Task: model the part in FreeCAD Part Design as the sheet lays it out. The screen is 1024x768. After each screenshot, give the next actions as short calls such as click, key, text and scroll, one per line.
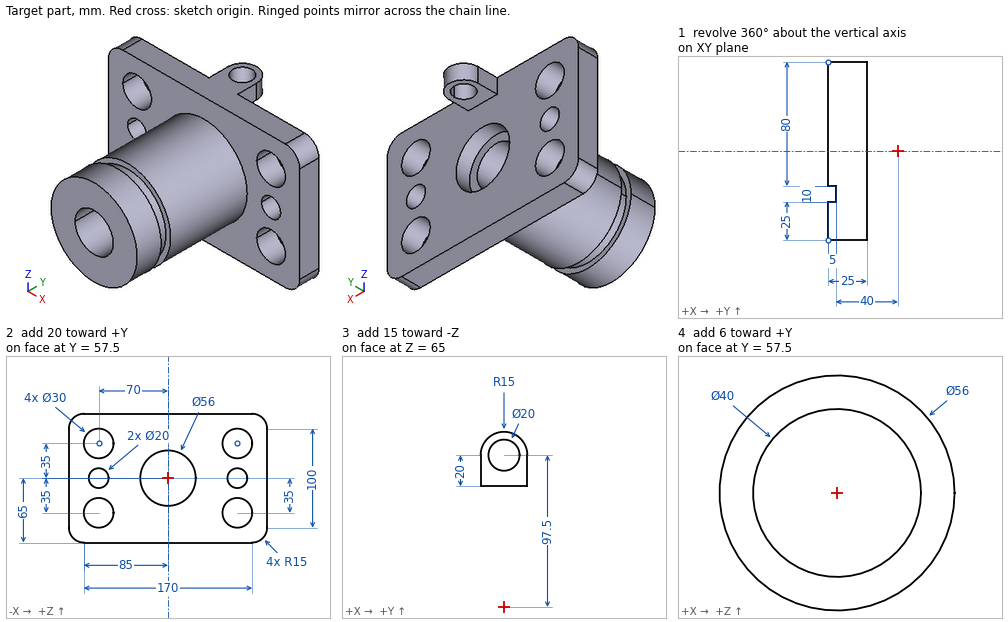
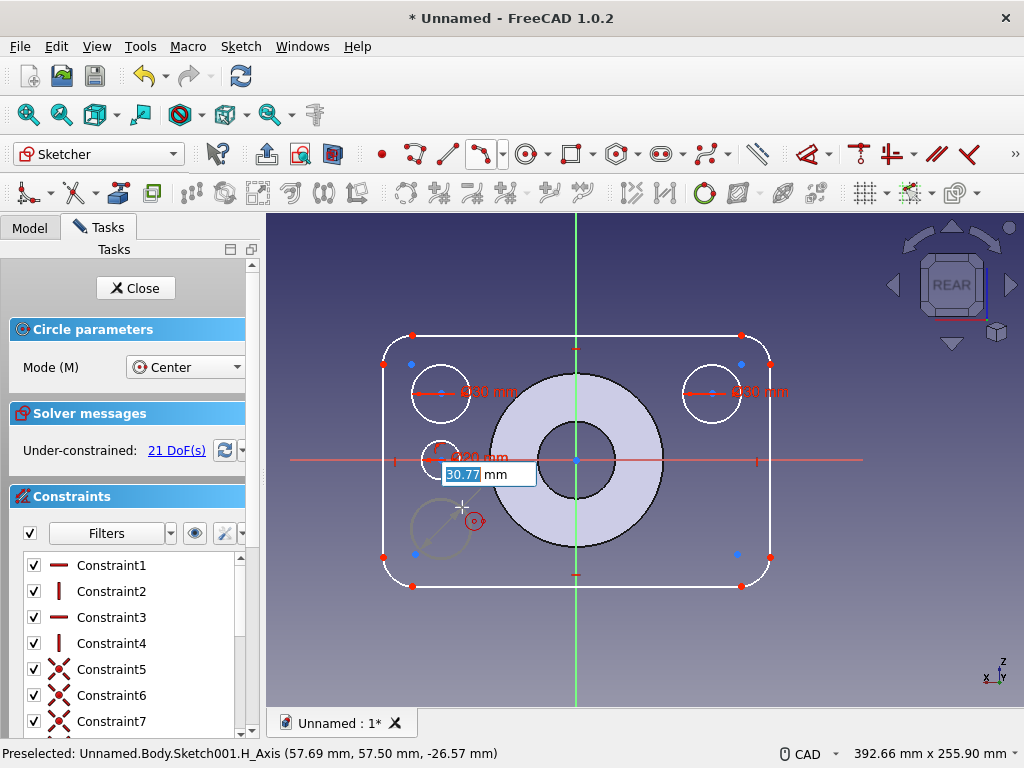
text(30)
key(Return)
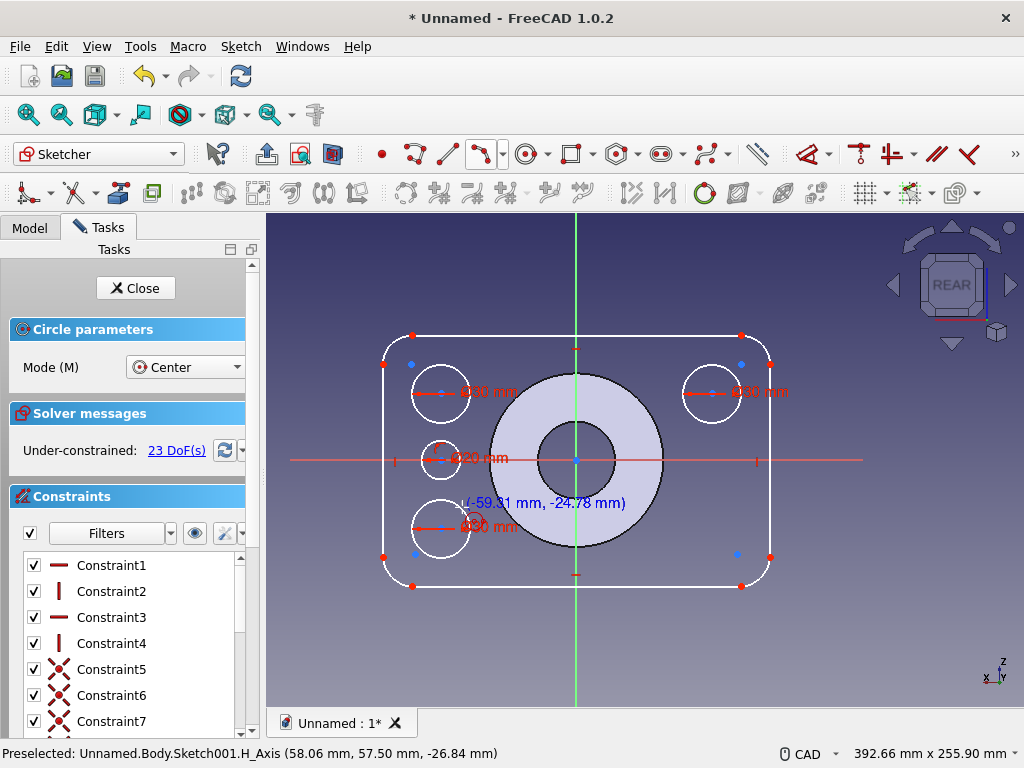
click(712, 460)
move(718, 442)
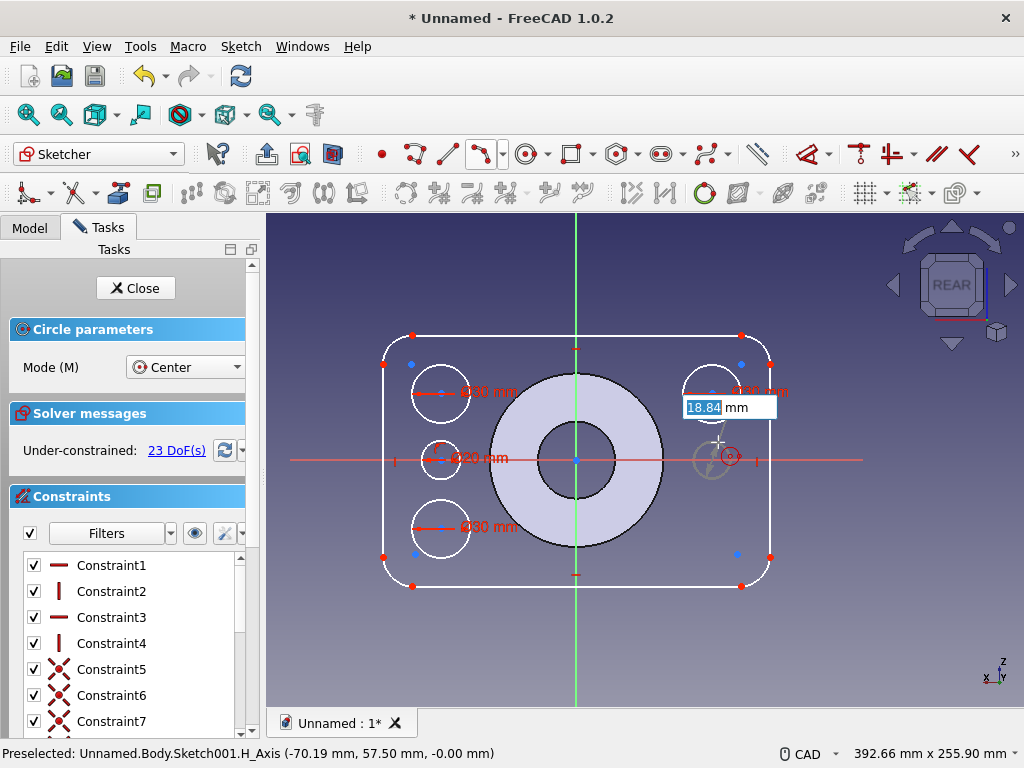
text(20)
key(Return)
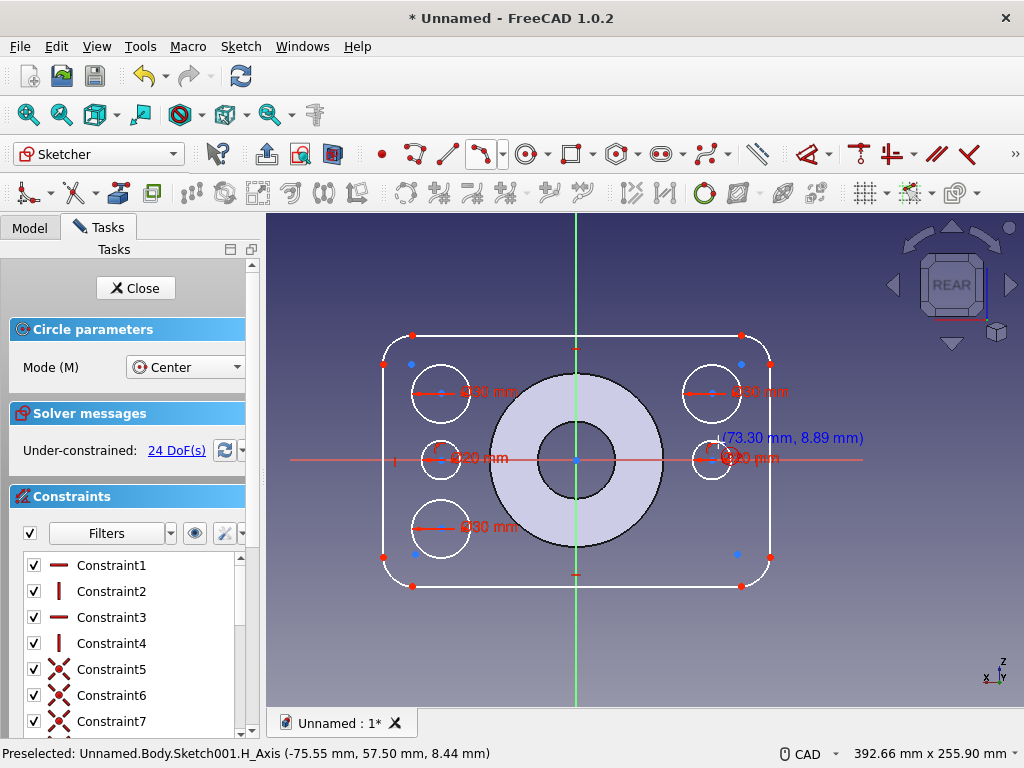
click(712, 528)
move(732, 507)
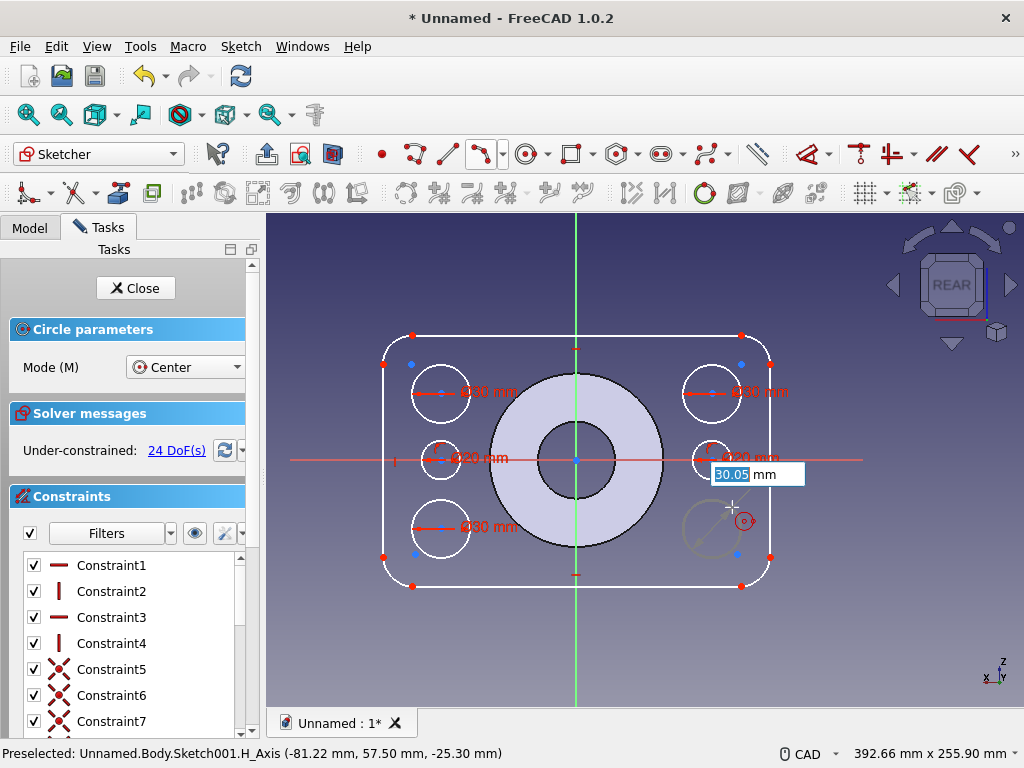
text(30)
key(Return)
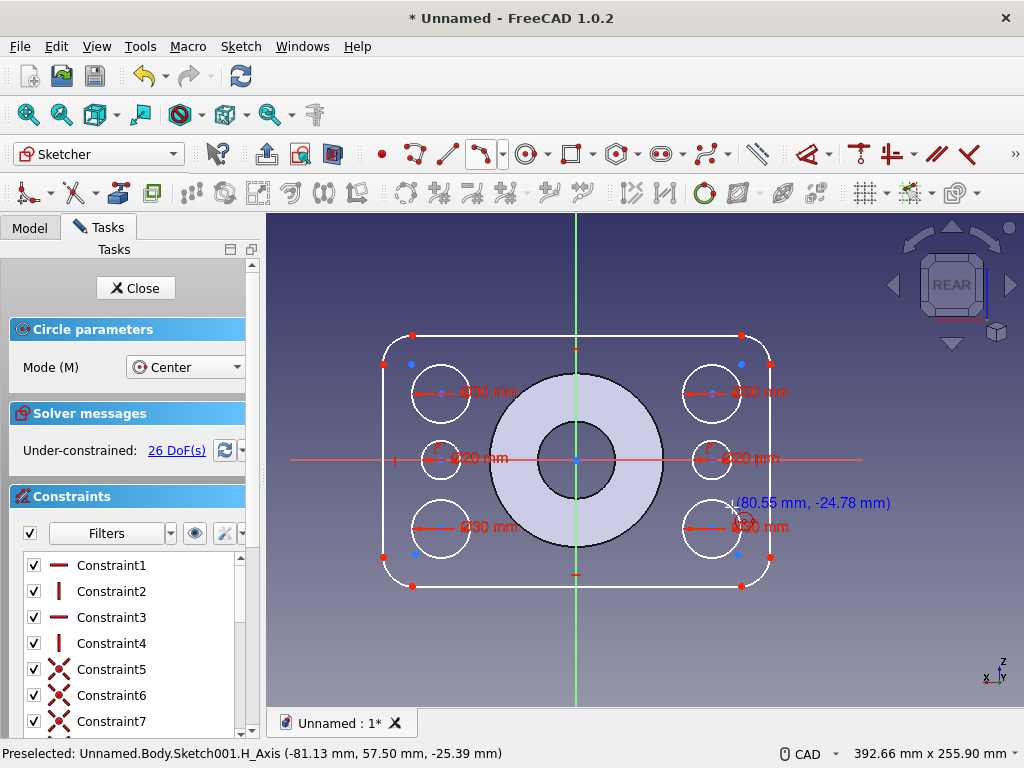
click(577, 460)
move(615, 422)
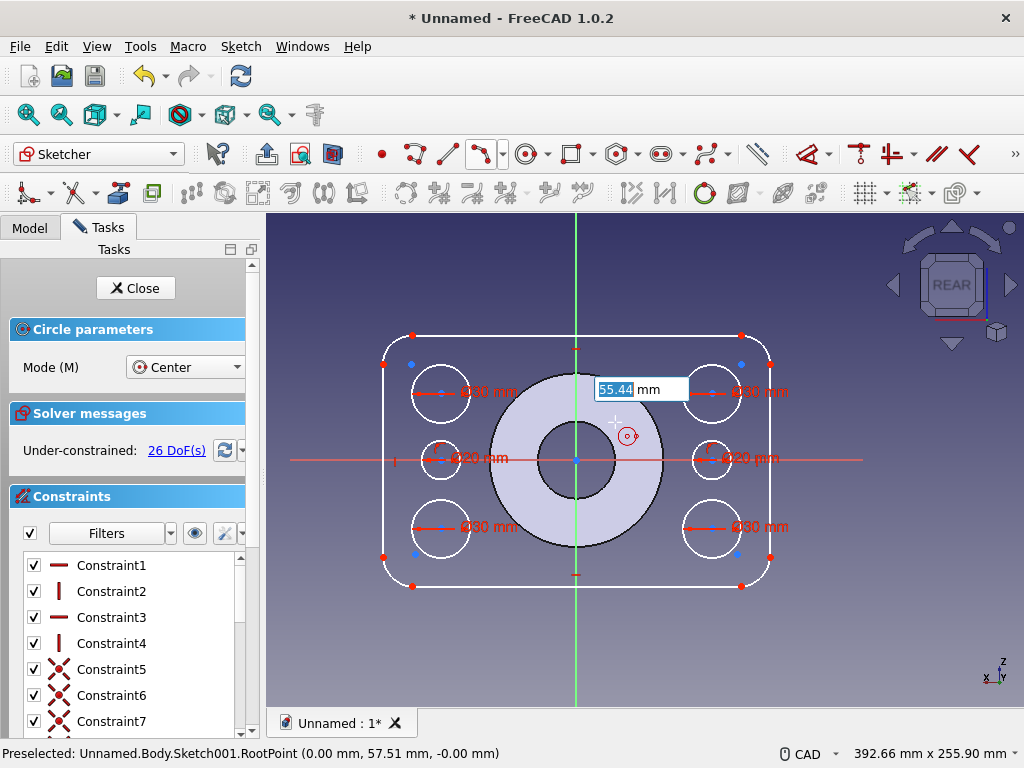
text(56)
key(Return)
key(Escape)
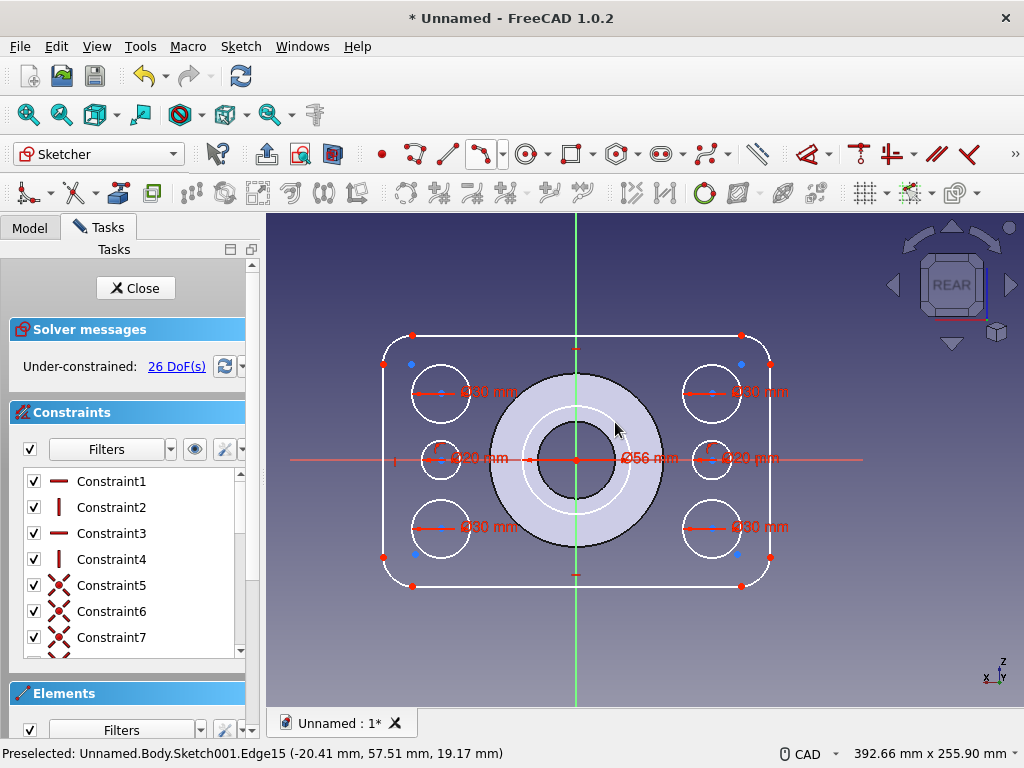
click(511, 587)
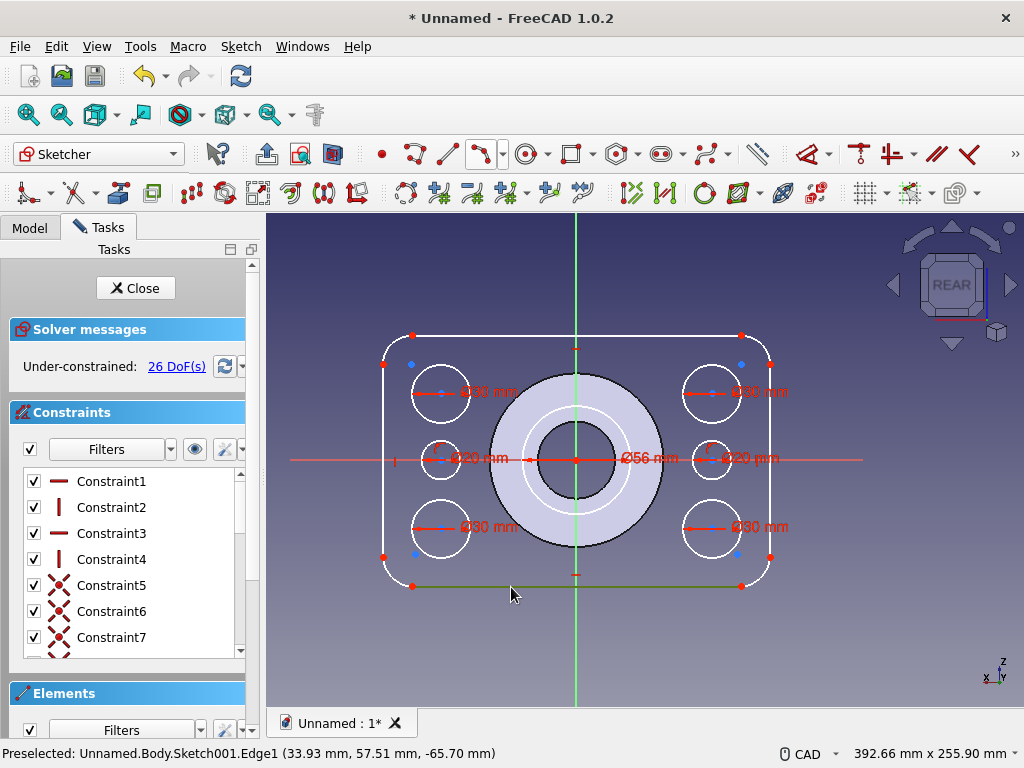
click(754, 583)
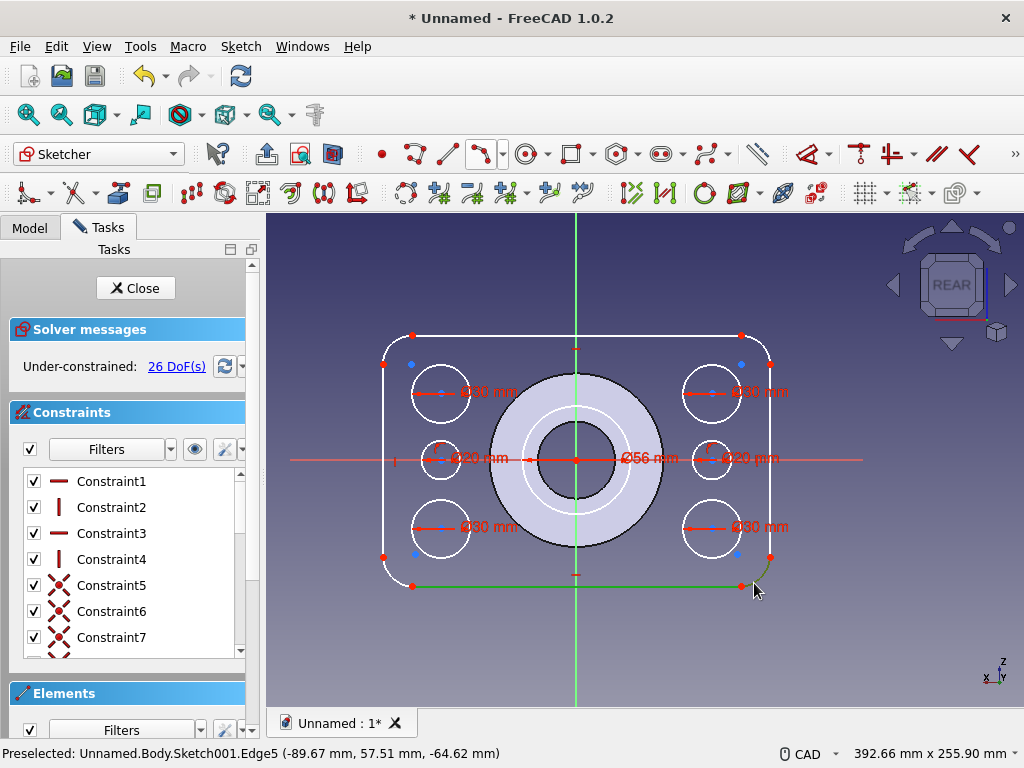
key(t)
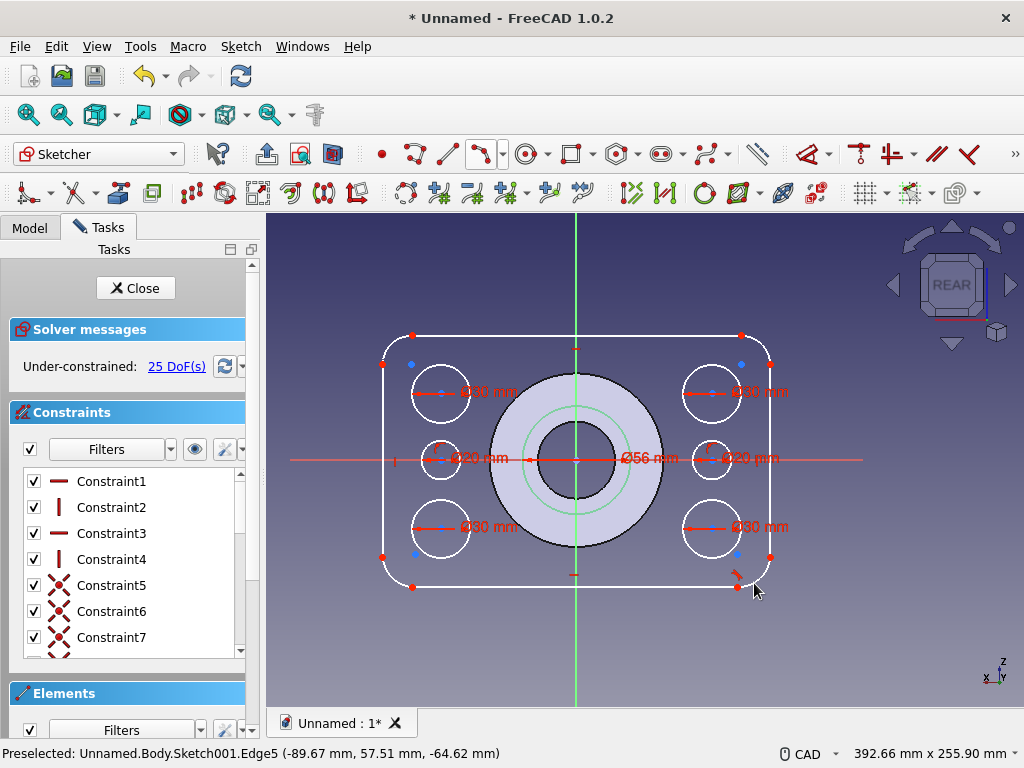
click(510, 587)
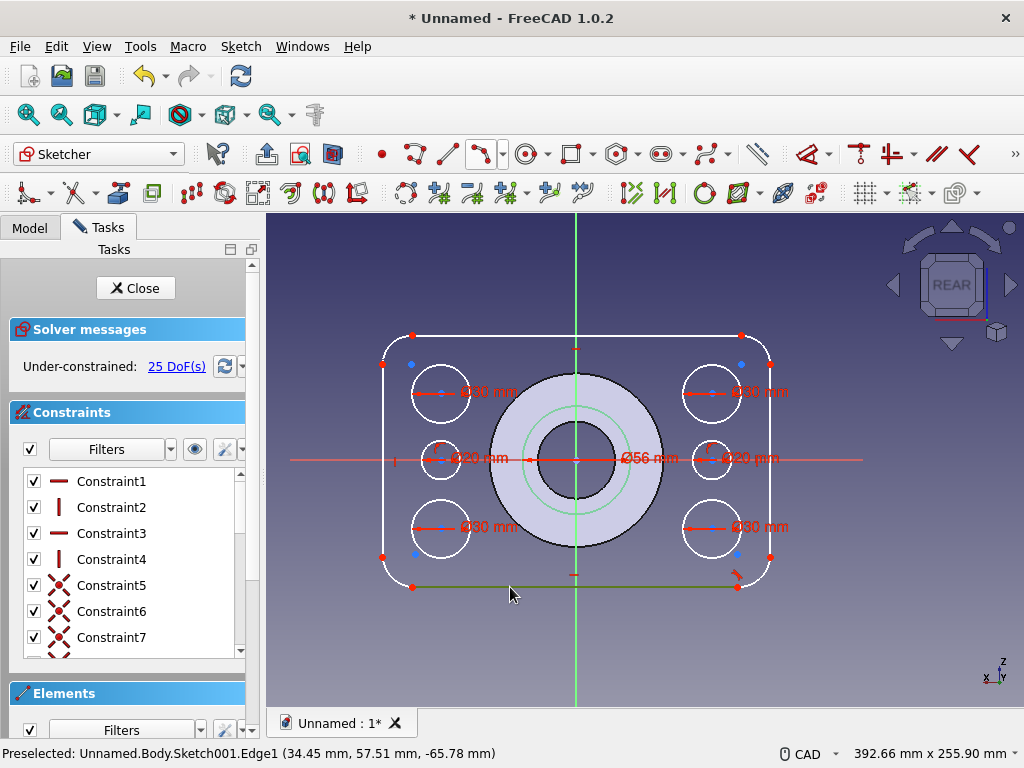
click(387, 571)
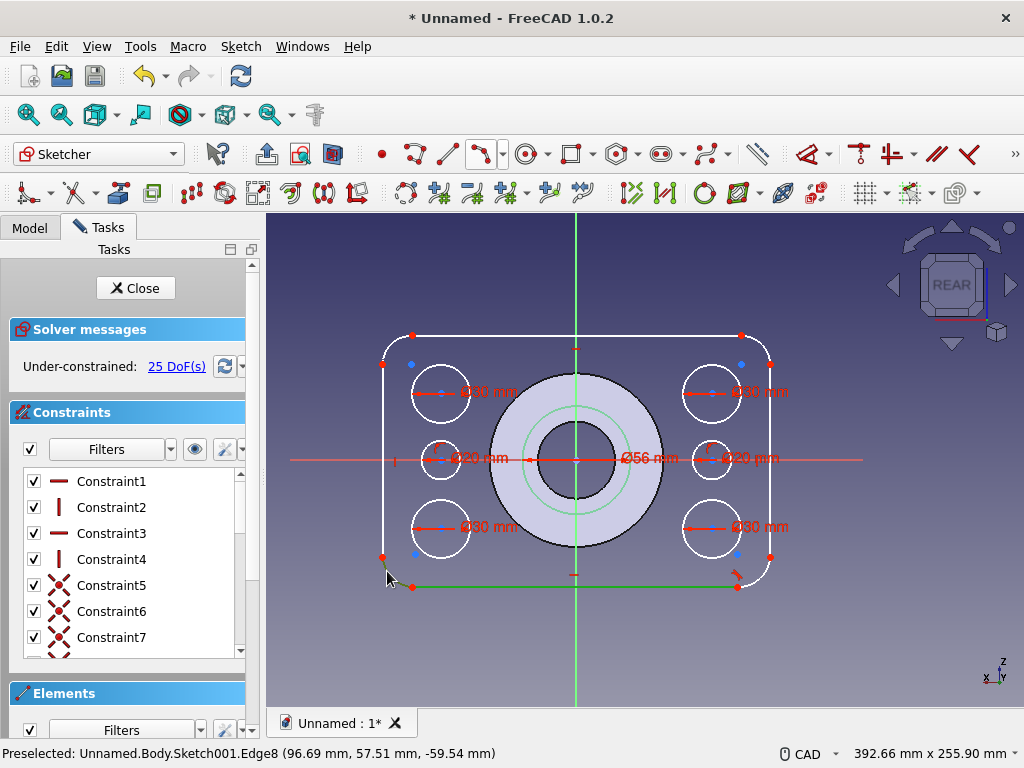
key(t)